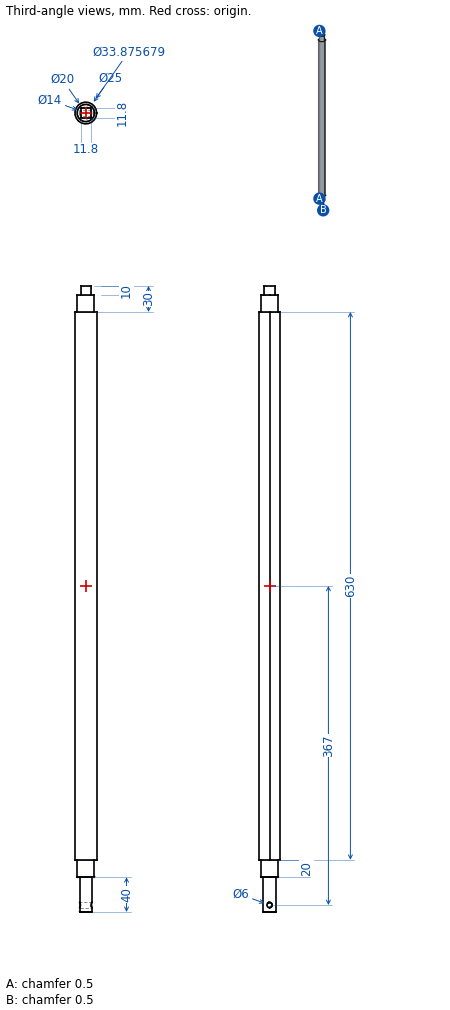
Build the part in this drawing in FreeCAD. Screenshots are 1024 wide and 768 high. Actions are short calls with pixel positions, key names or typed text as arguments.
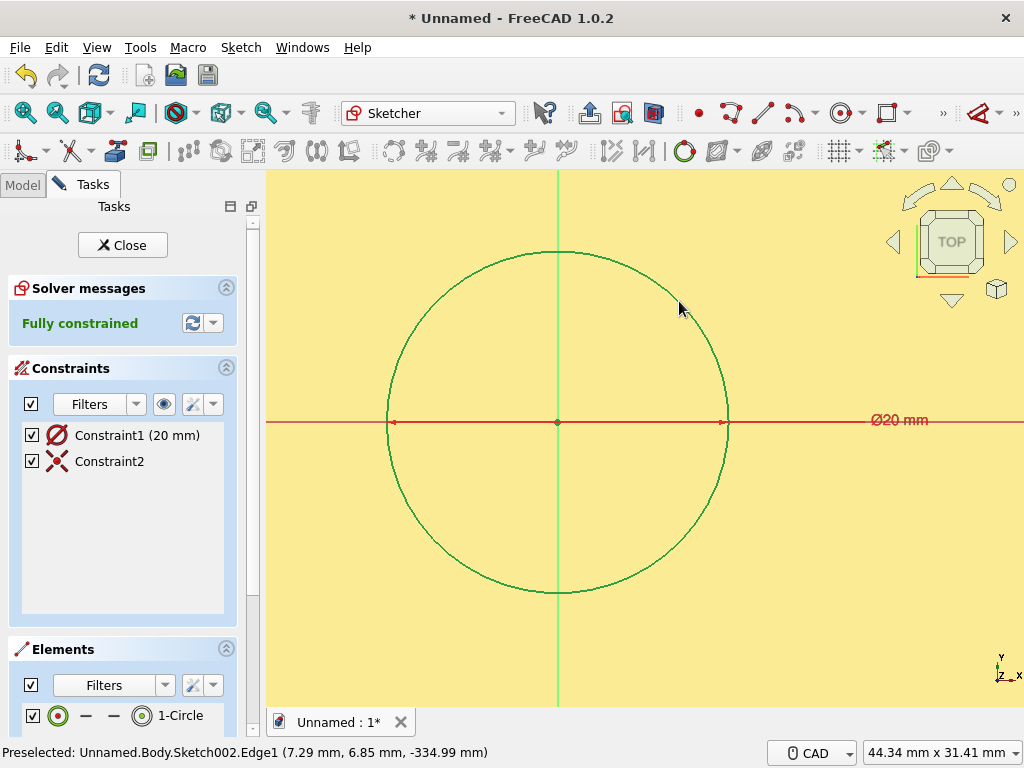
click(123, 245)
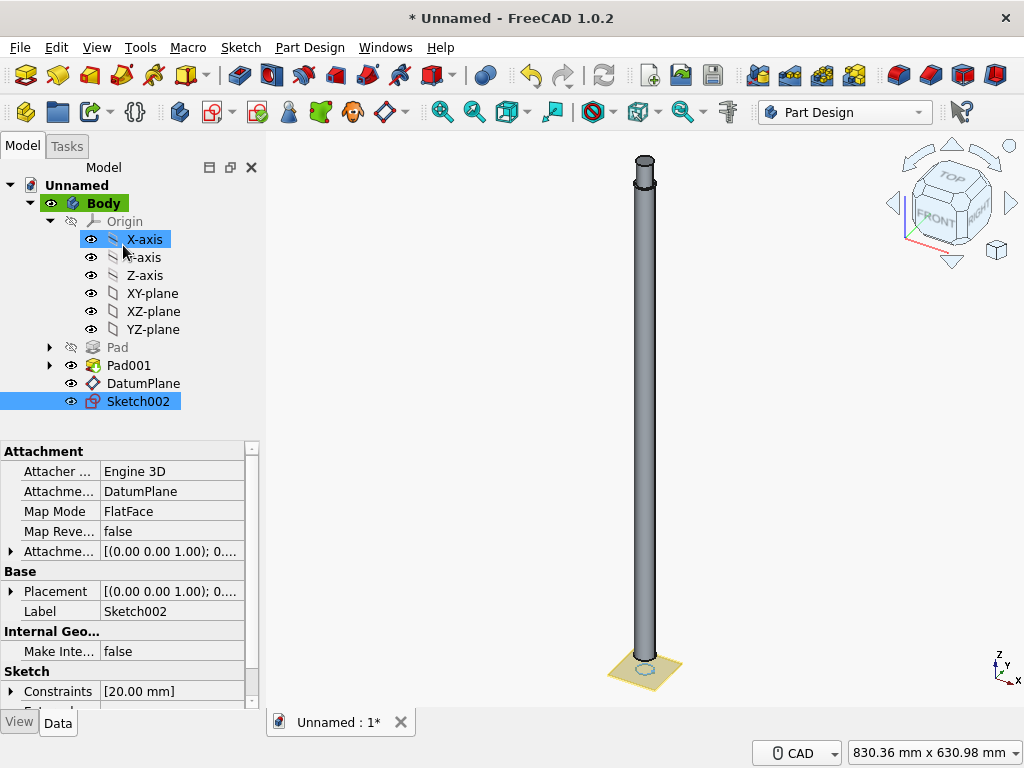
click(26, 76)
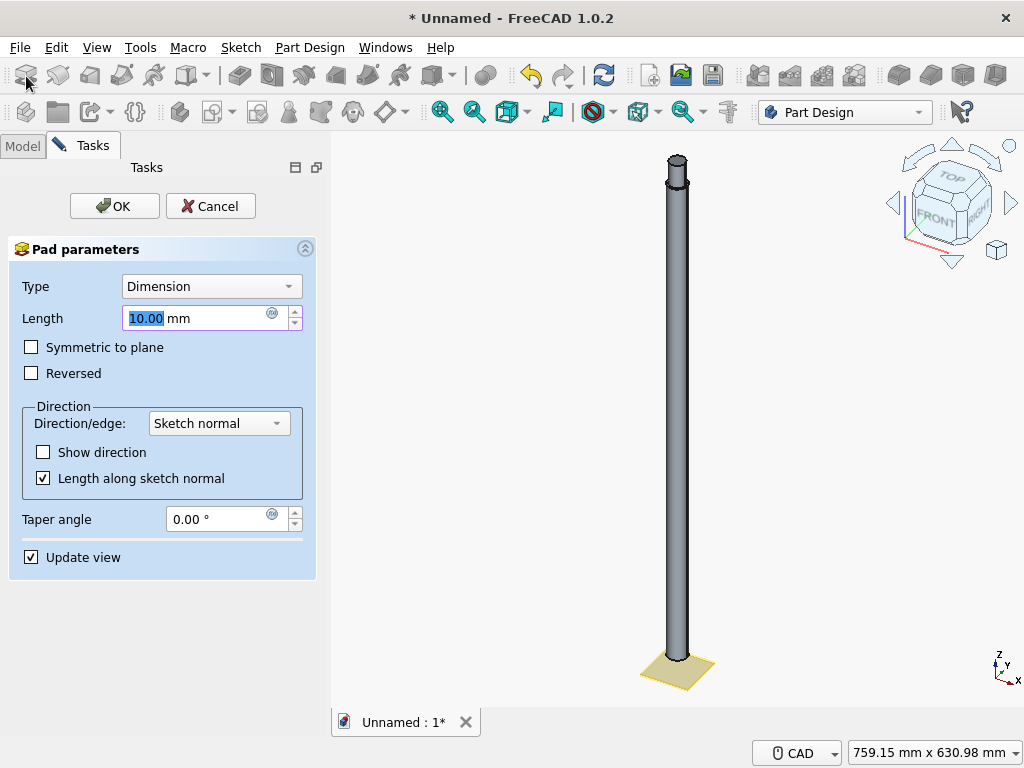
text(20)
key(Tab)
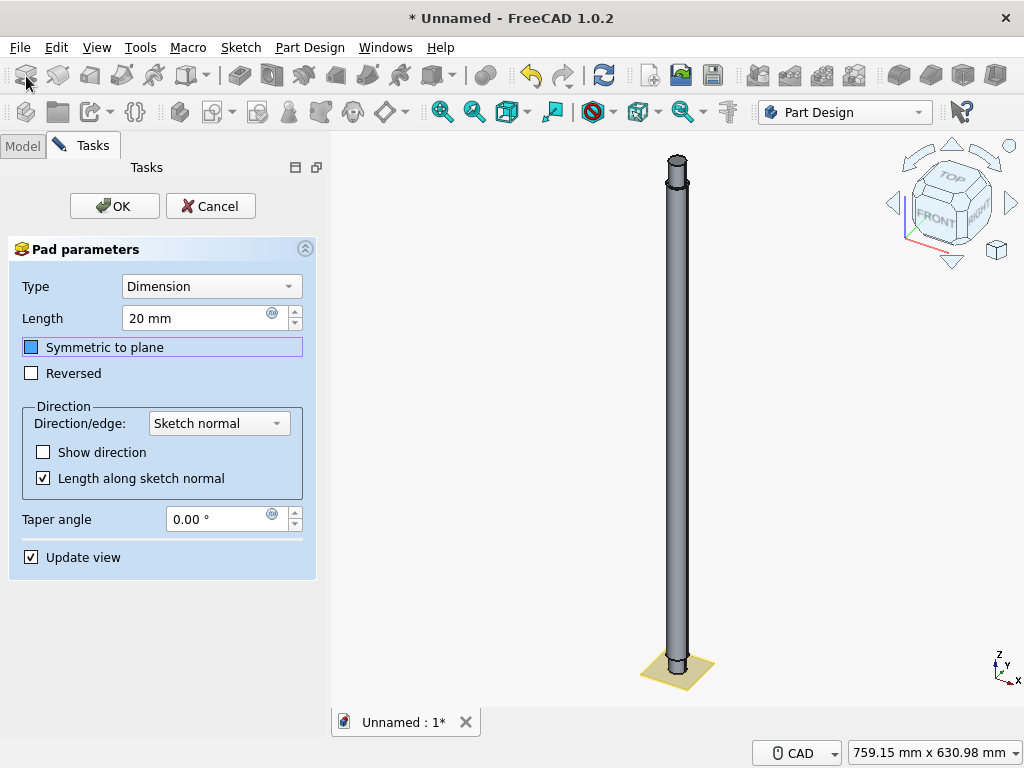
click(115, 206)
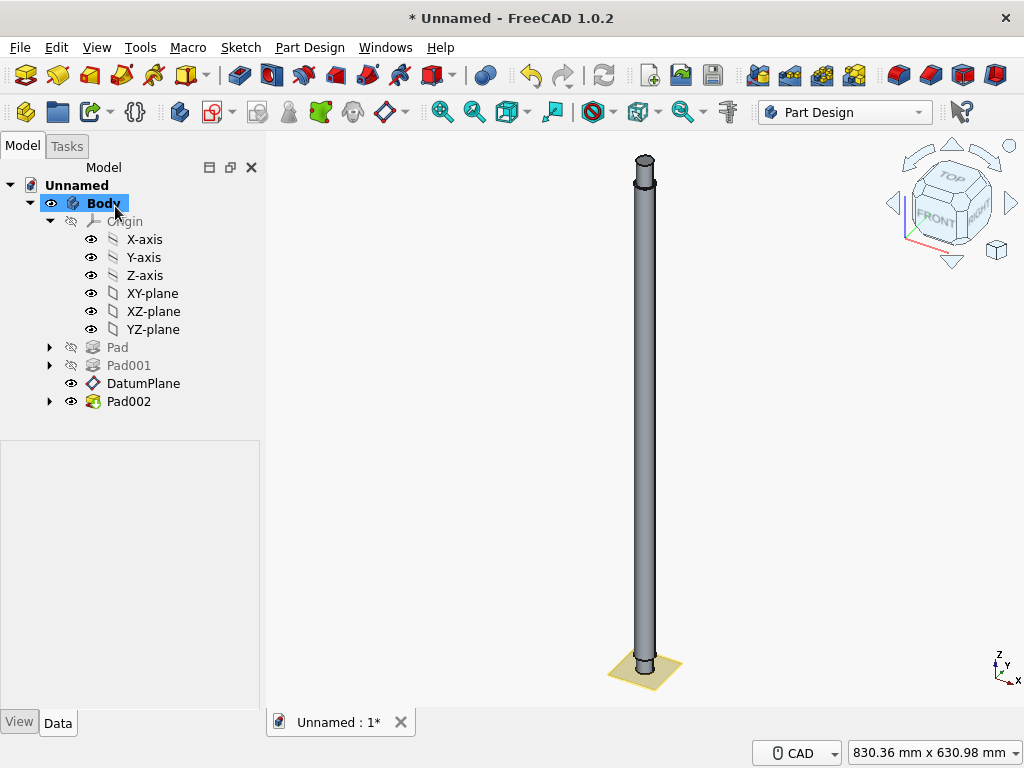
click(116, 383)
key(space)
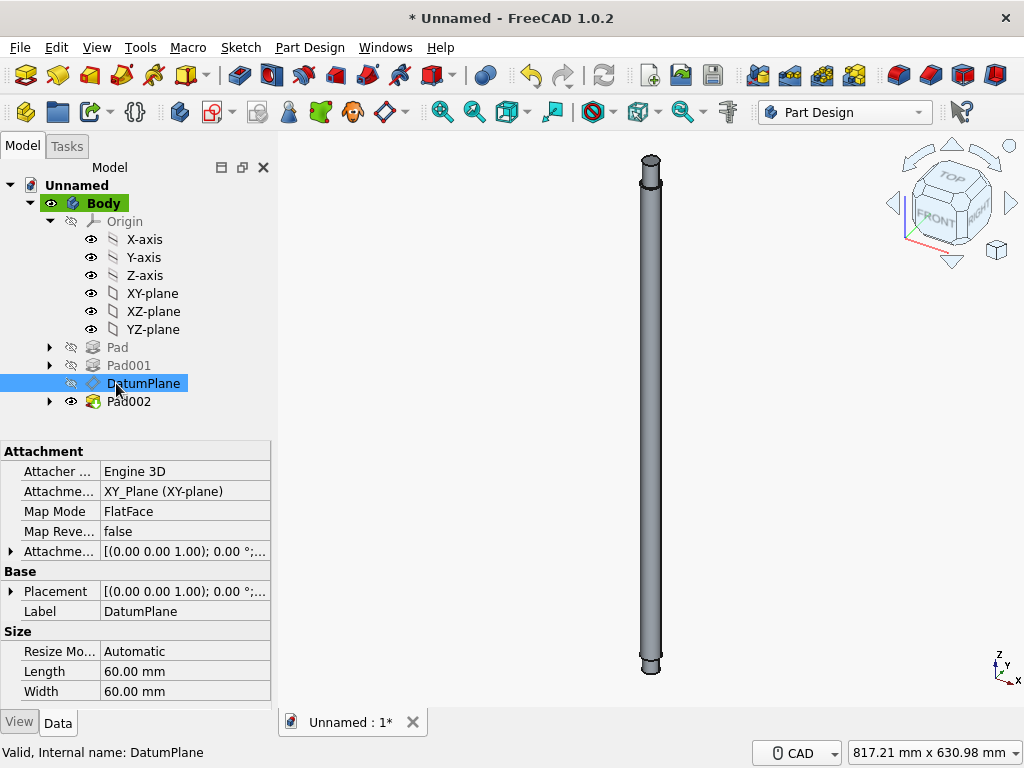
click(644, 672)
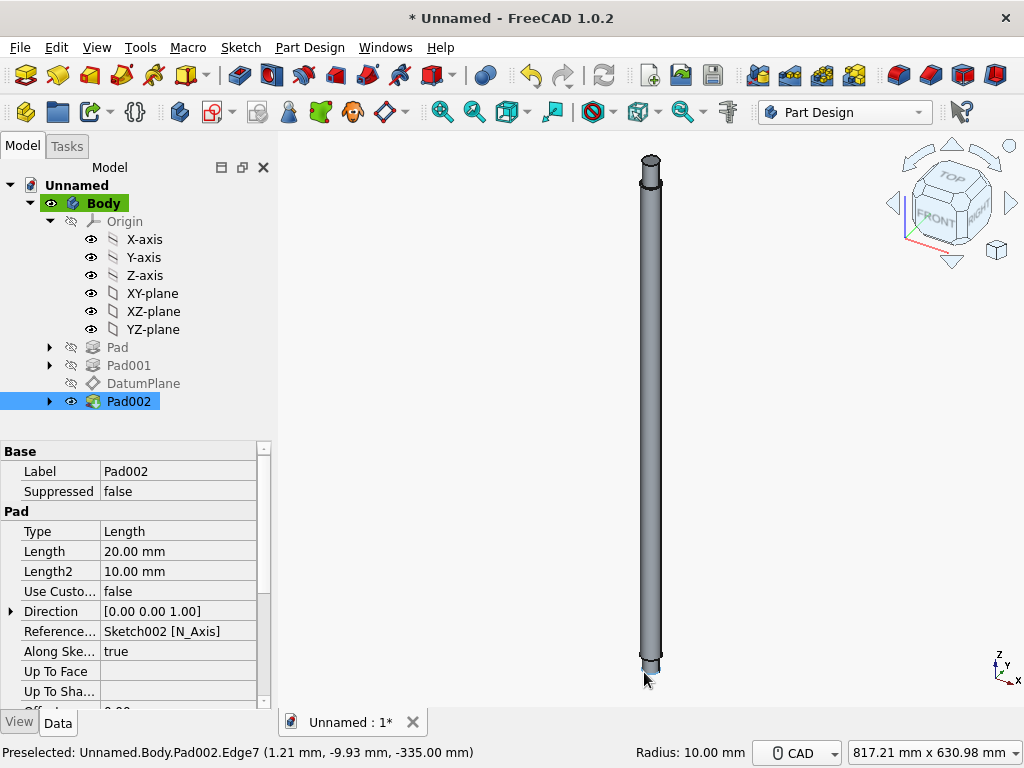
click(642, 160, ctrl)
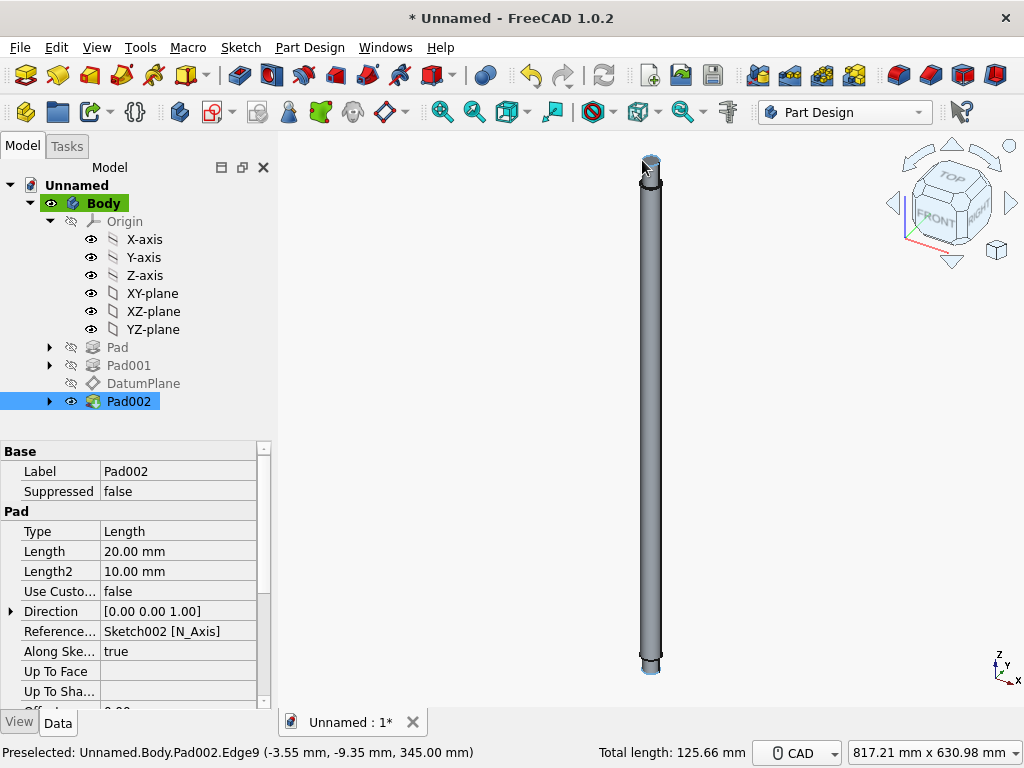
click(932, 76)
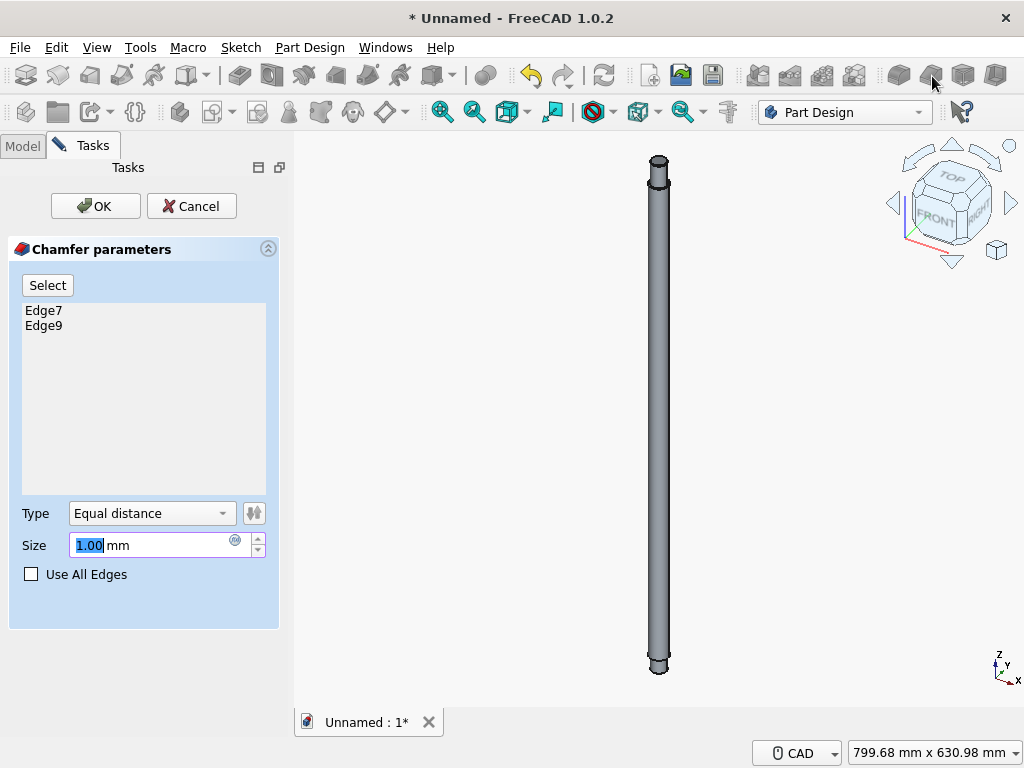
text(0.5)
key(Tab)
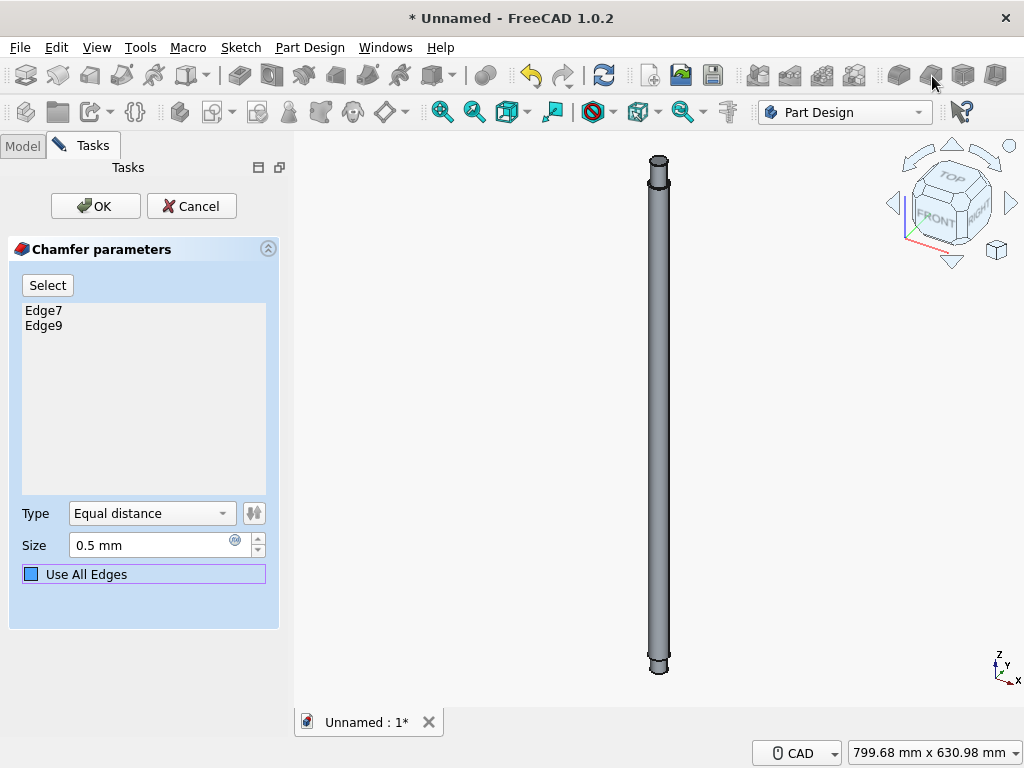
click(96, 206)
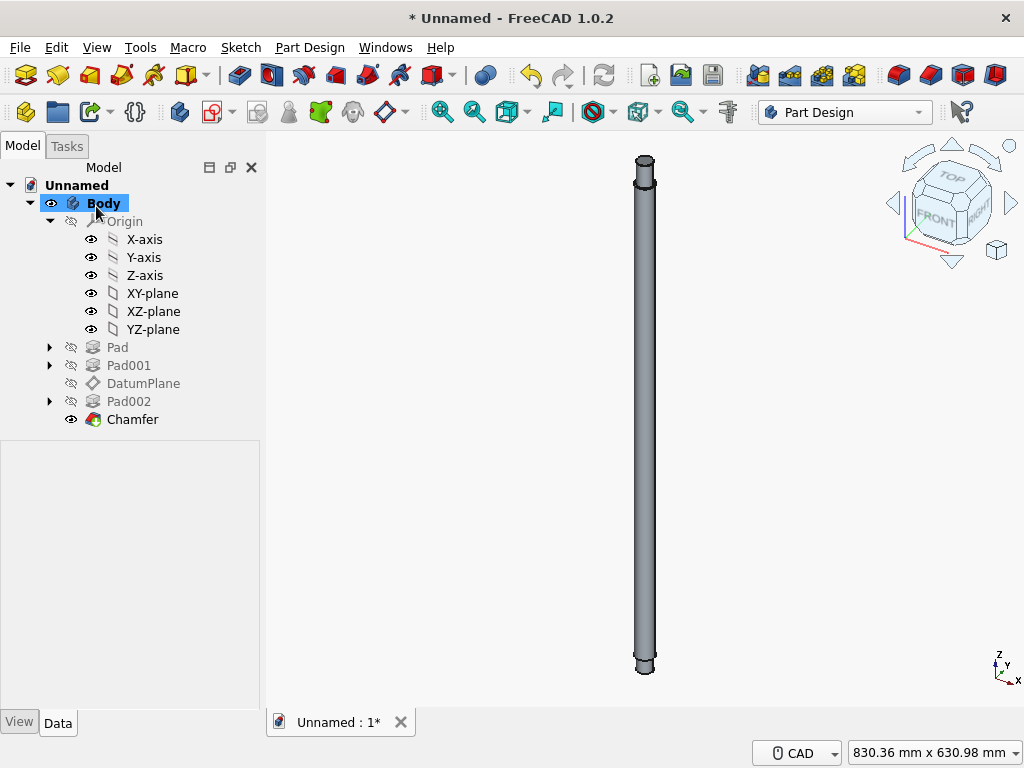
key(5)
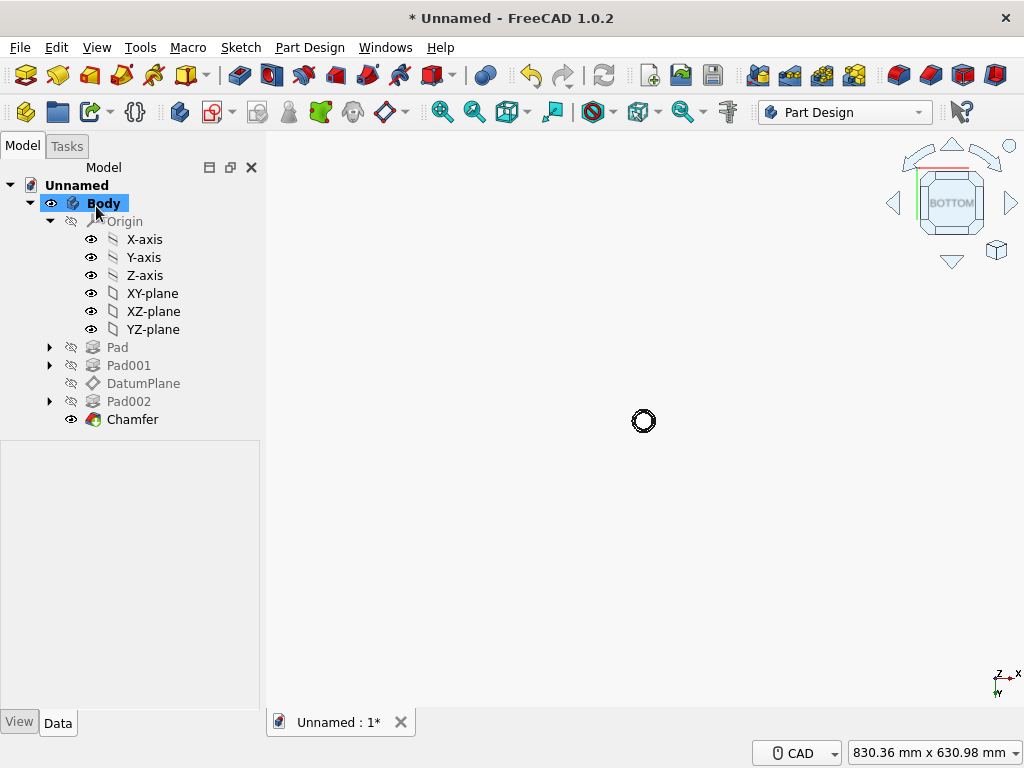
click(444, 112)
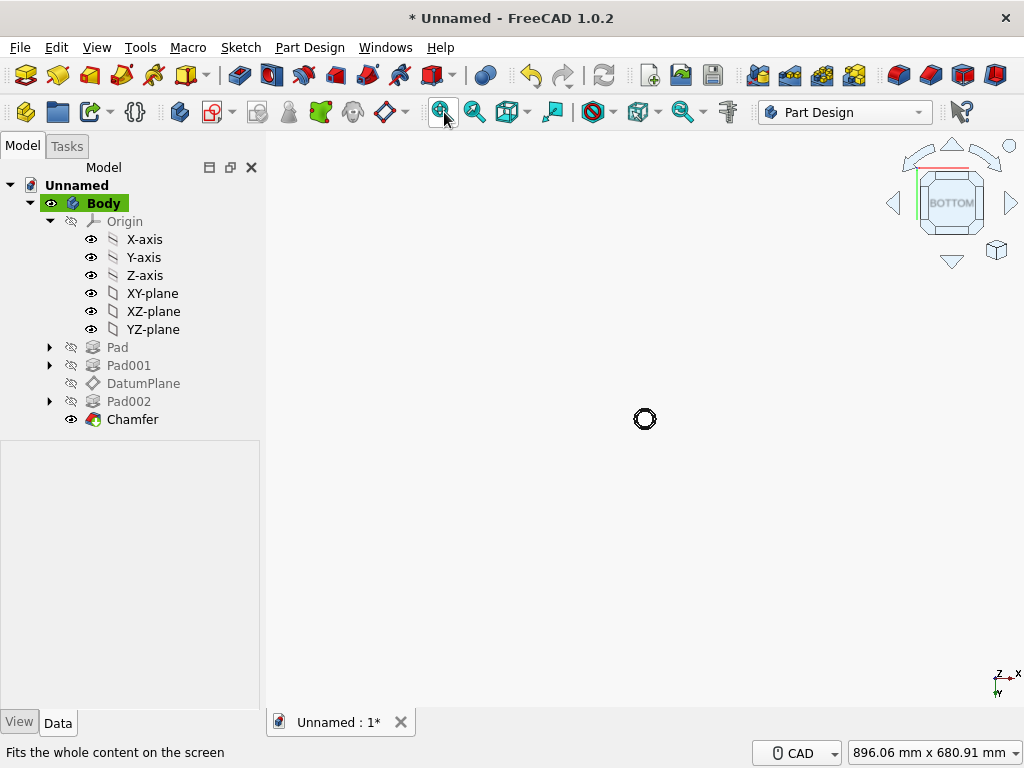
key(1)